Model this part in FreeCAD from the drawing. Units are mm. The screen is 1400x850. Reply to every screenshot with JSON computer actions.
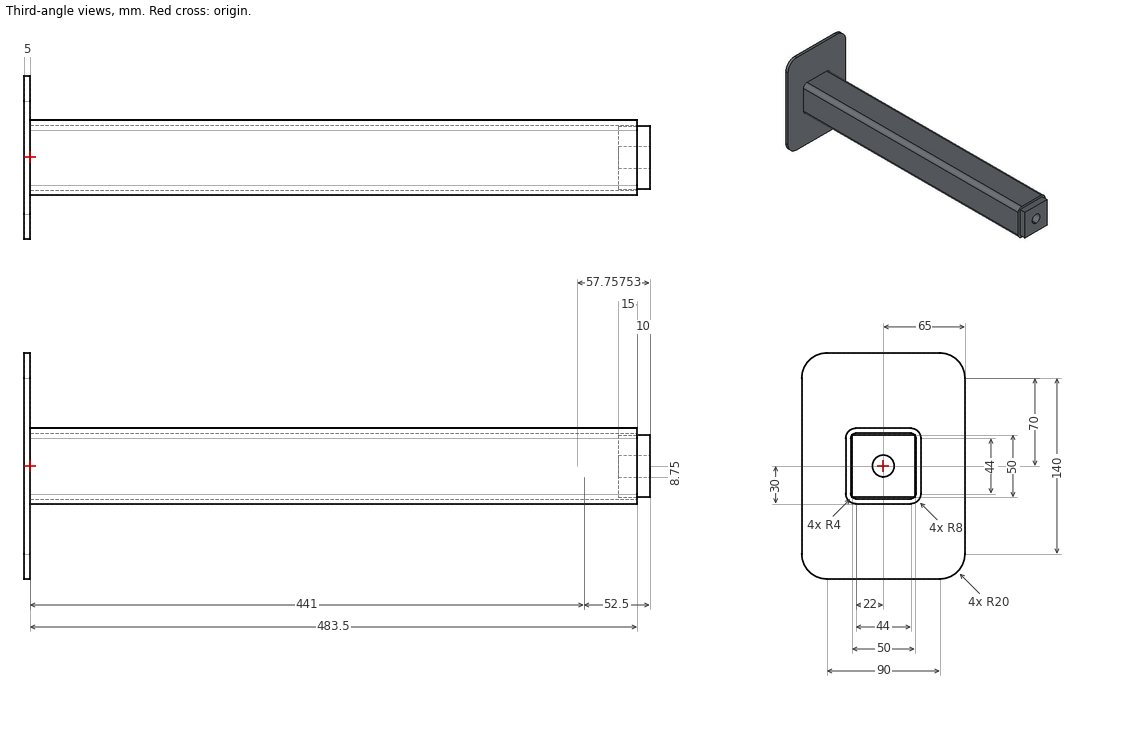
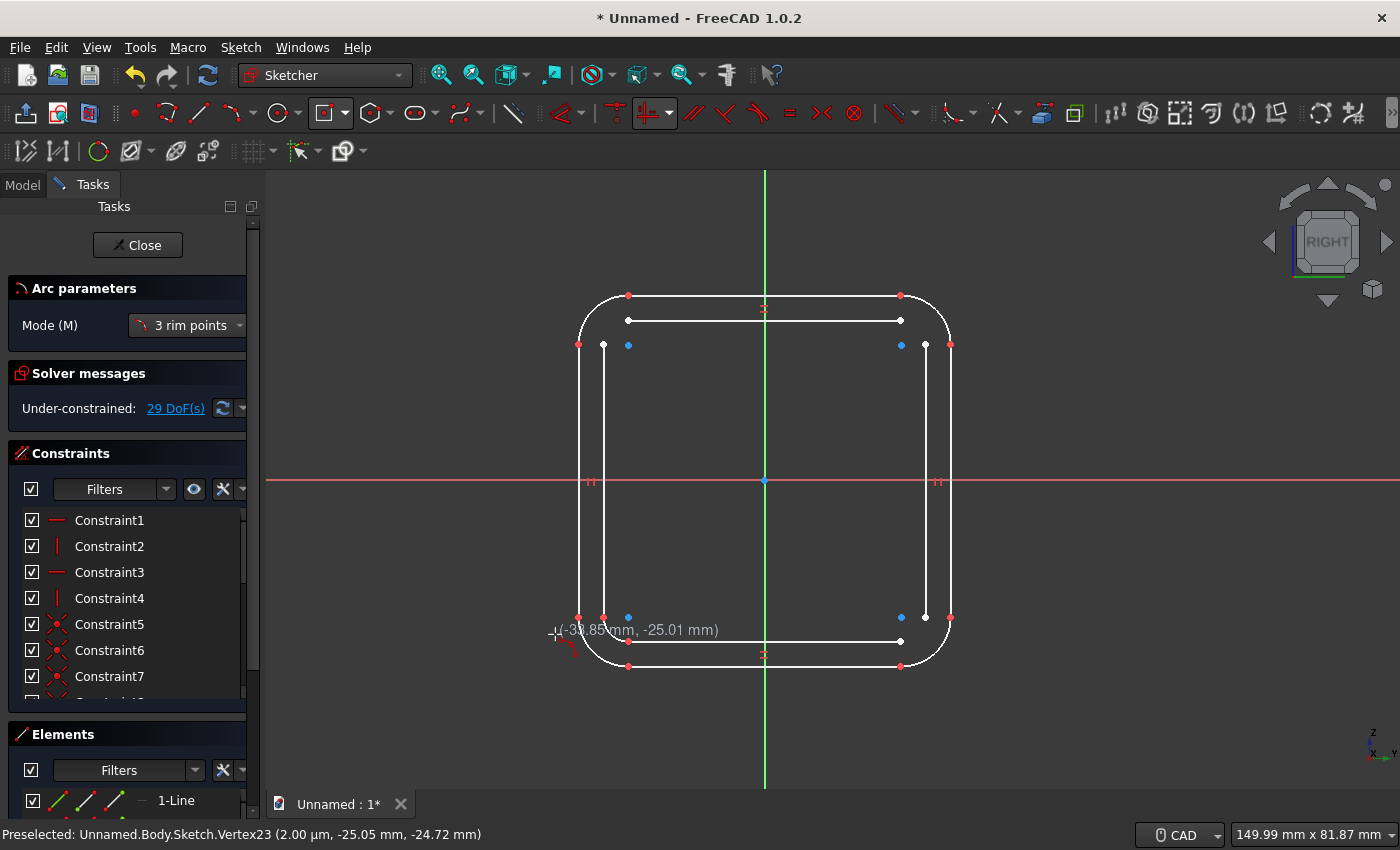
{"action": "left_click", "coordinate": [604, 345]}
{"action": "left_click", "coordinate": [629, 321]}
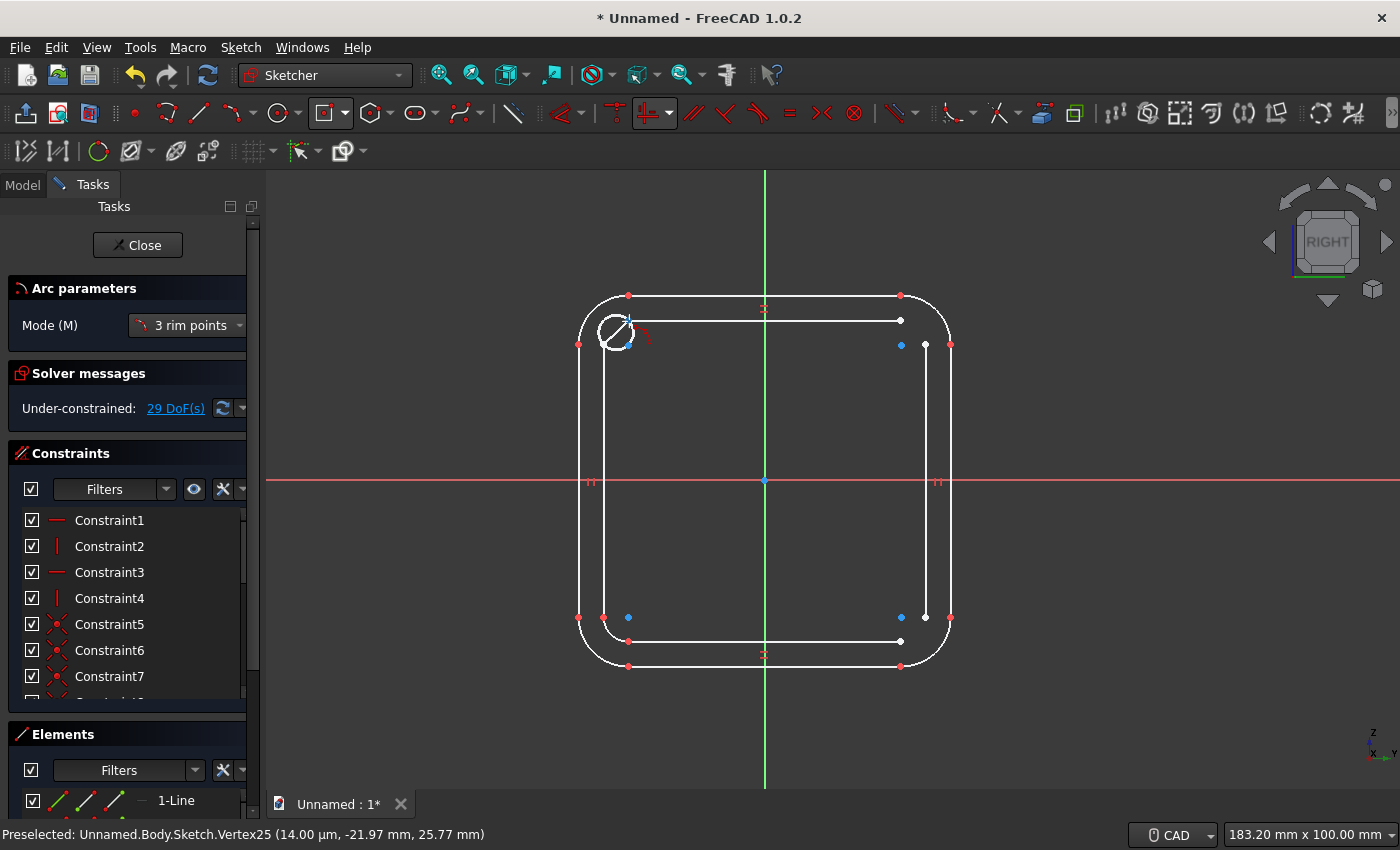
{"action": "scroll", "coordinate": [611, 326], "scroll_direction": "up", "scroll_amount": 4}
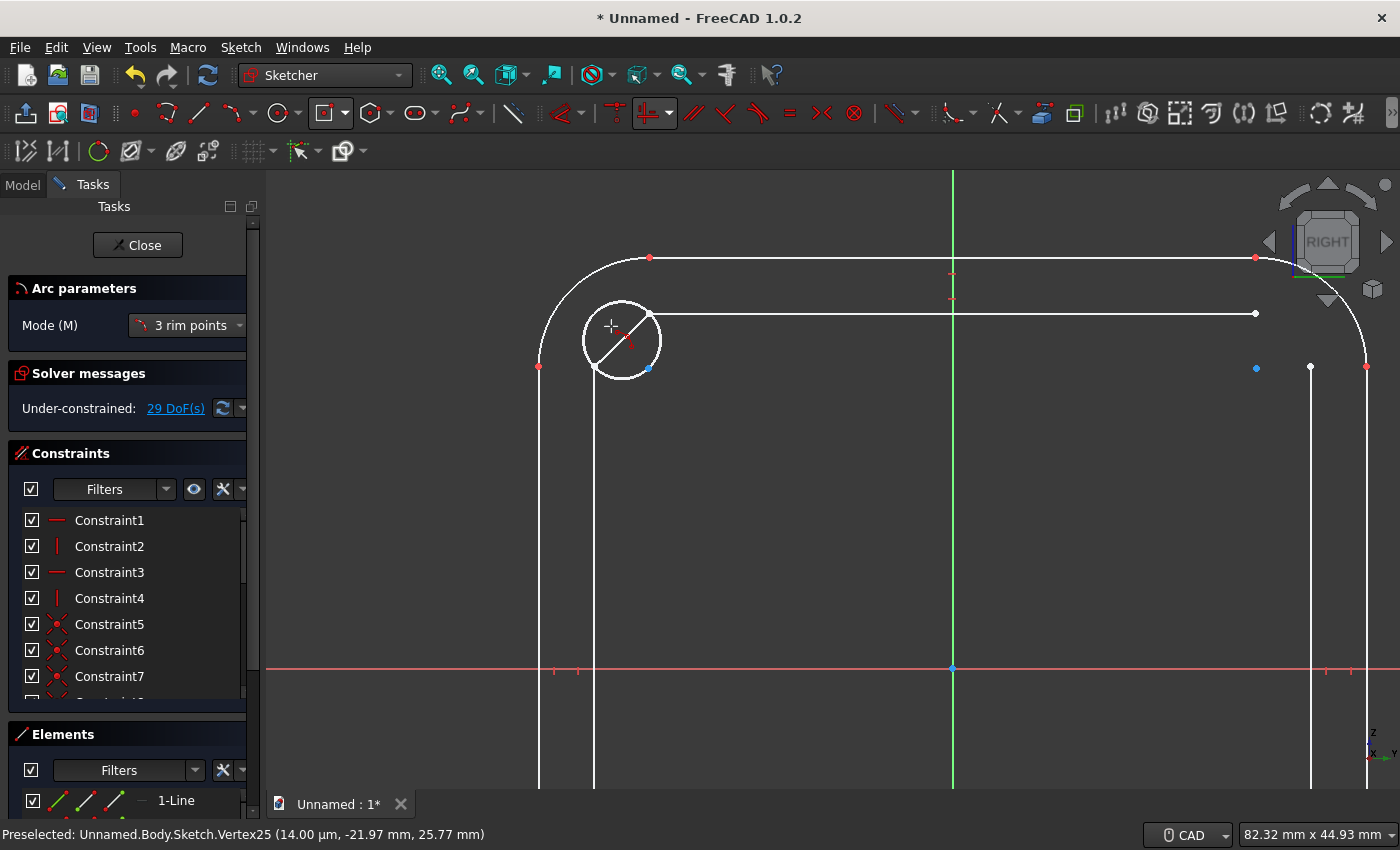
{"action": "left_click", "coordinate": [611, 327]}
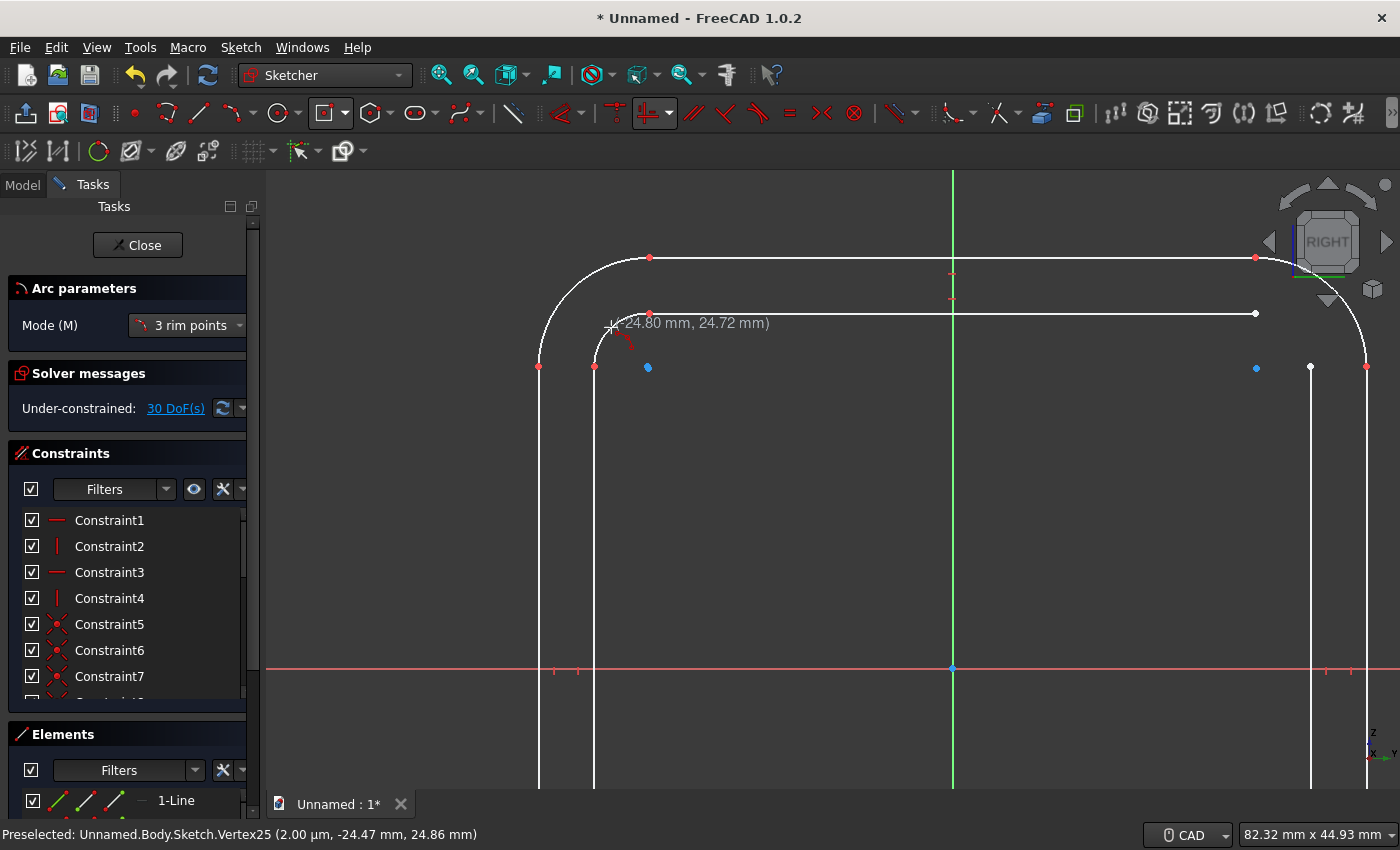
{"action": "scroll", "coordinate": [611, 325], "scroll_direction": "down", "scroll_amount": 4}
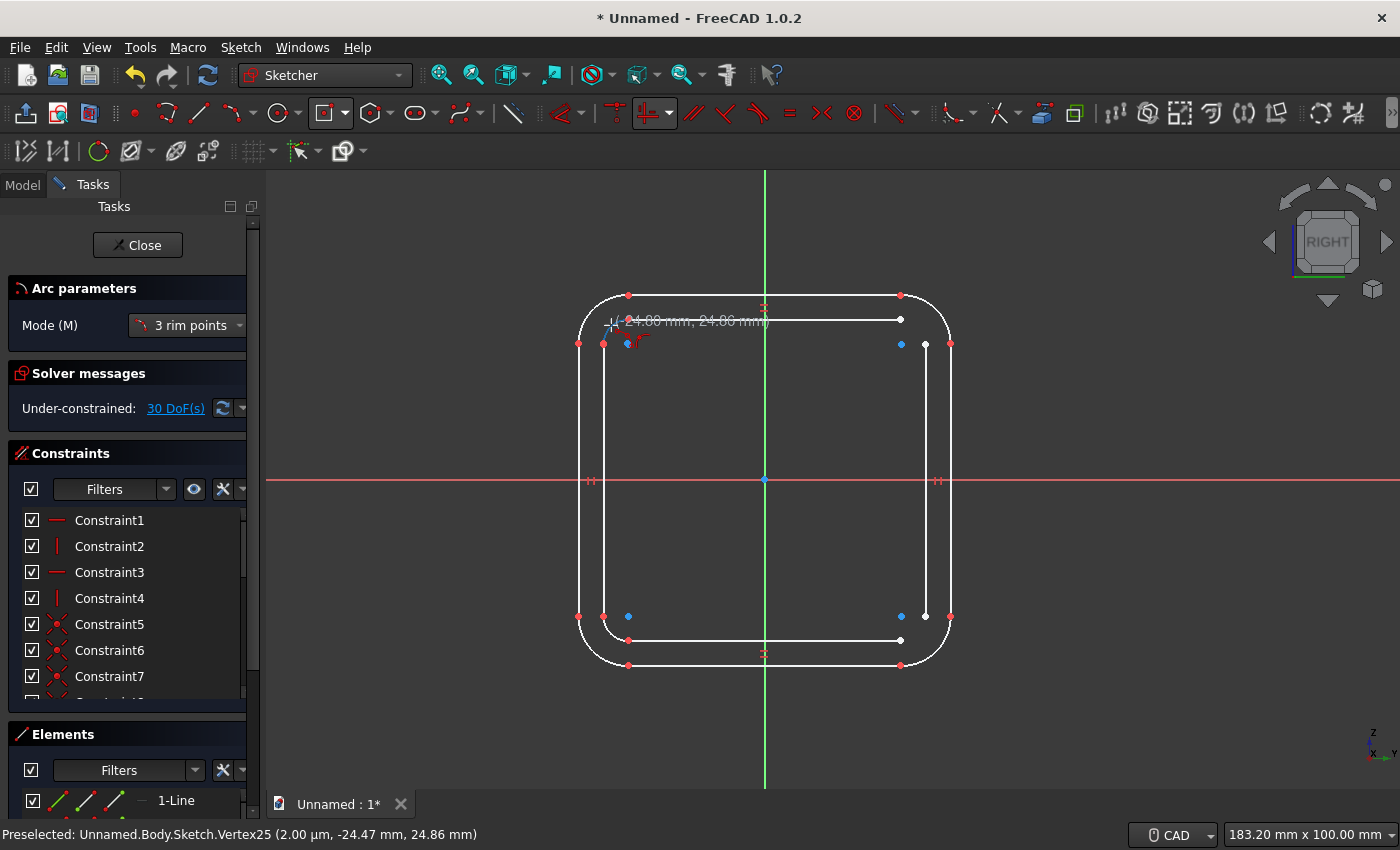
{"action": "left_click", "coordinate": [901, 320]}
{"action": "left_click", "coordinate": [926, 344]}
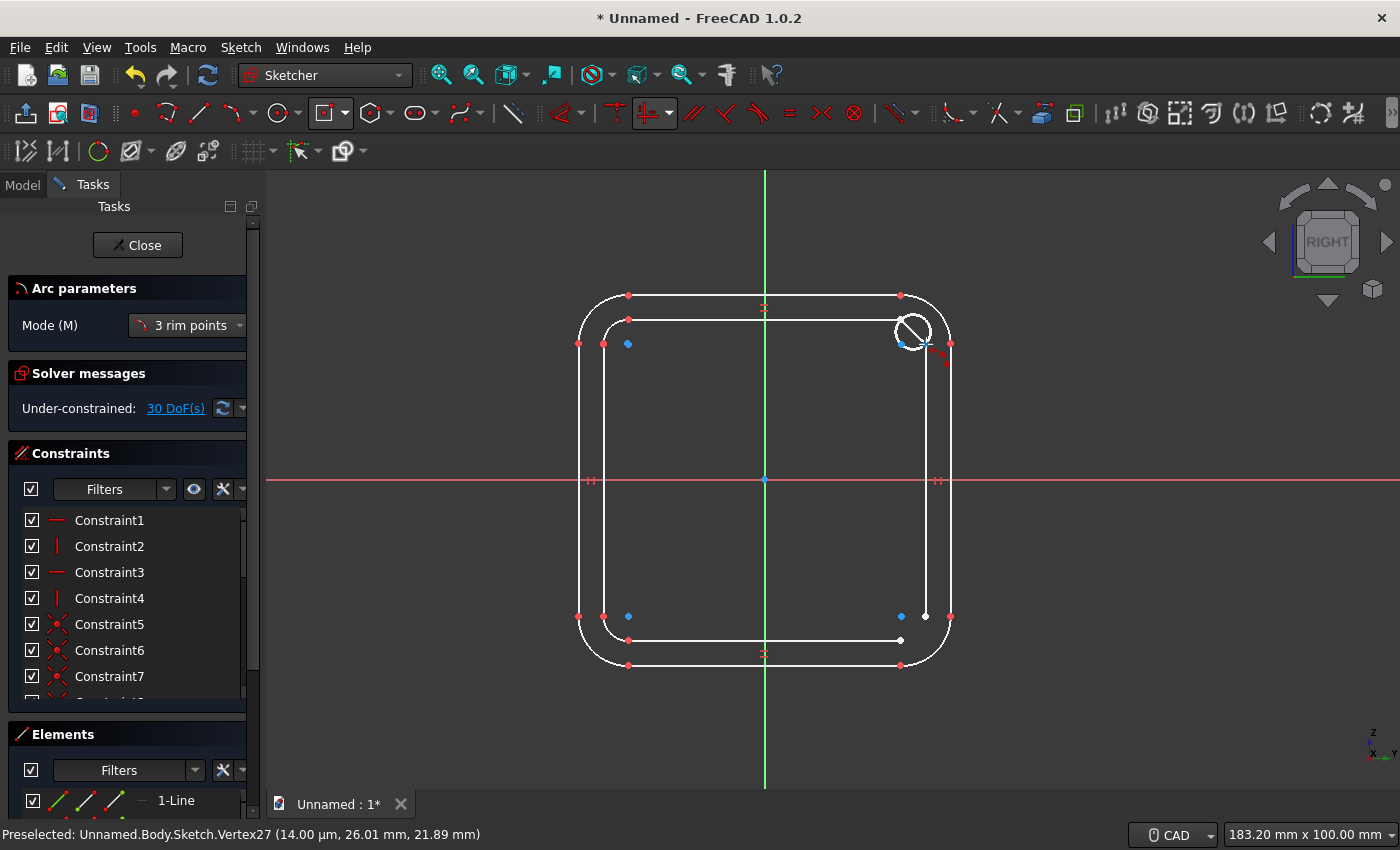
{"action": "scroll", "coordinate": [918, 326], "scroll_direction": "up", "scroll_amount": 4}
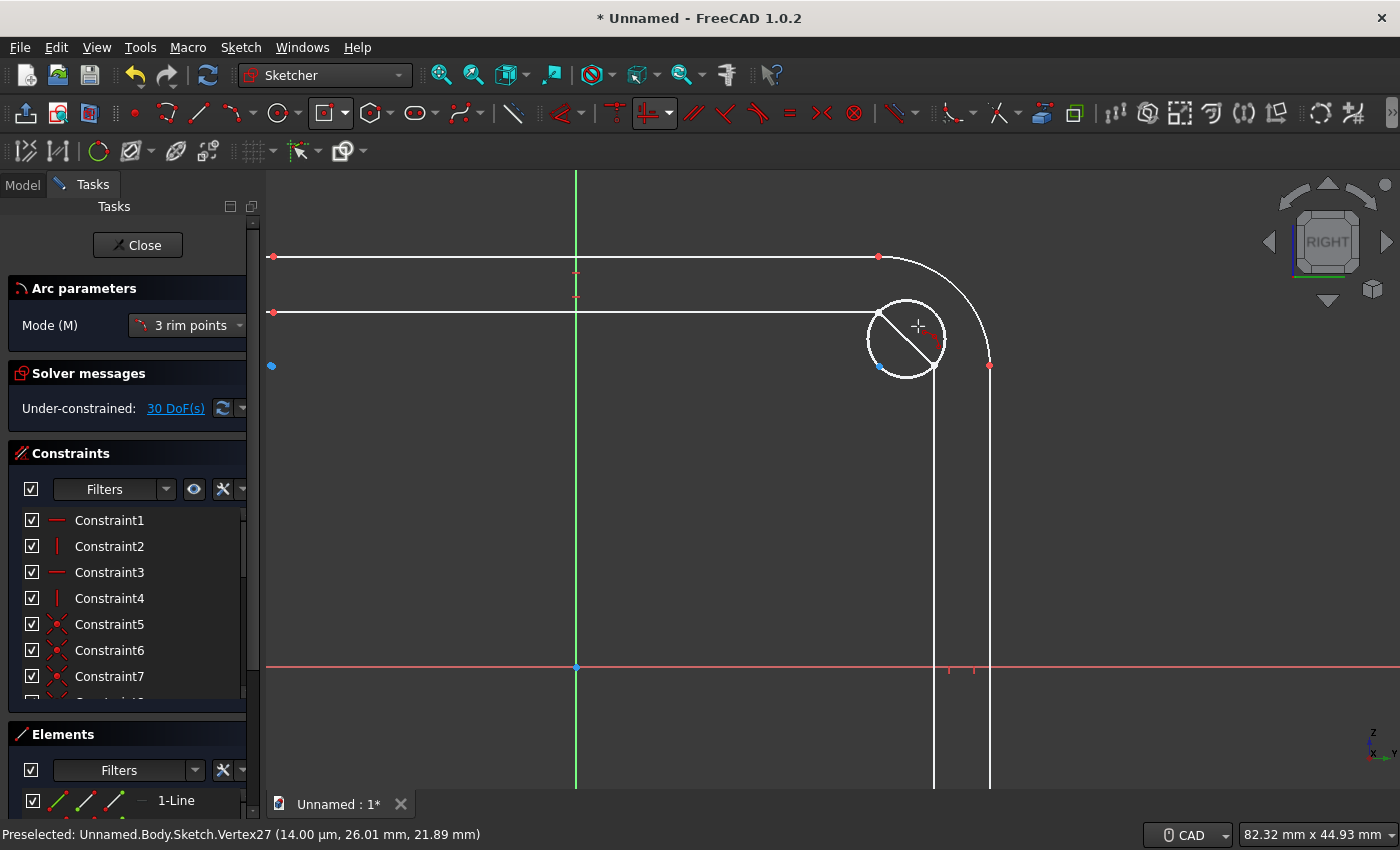
{"action": "left_click", "coordinate": [918, 325]}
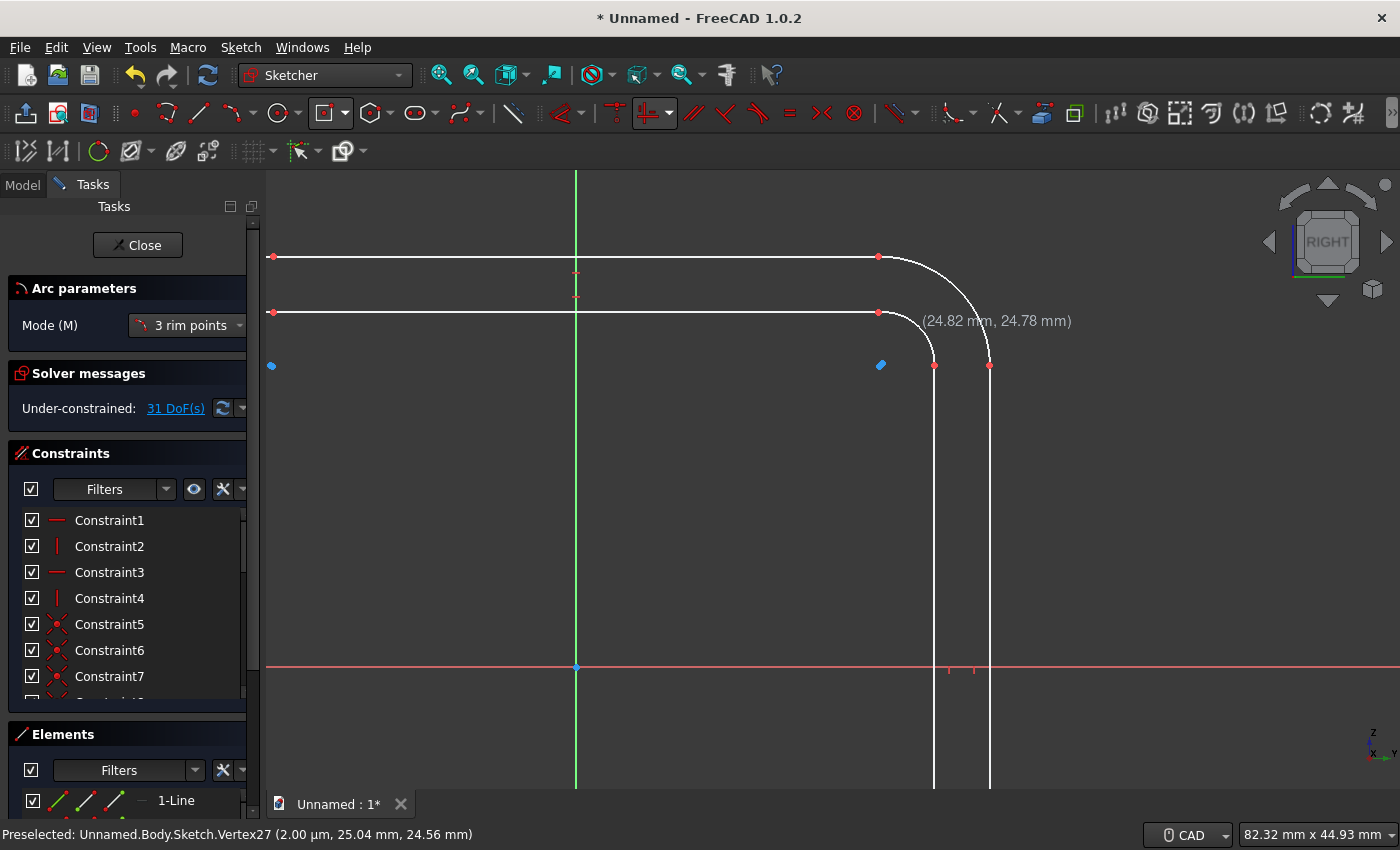
{"action": "scroll", "coordinate": [918, 326], "scroll_direction": "down", "scroll_amount": 4}